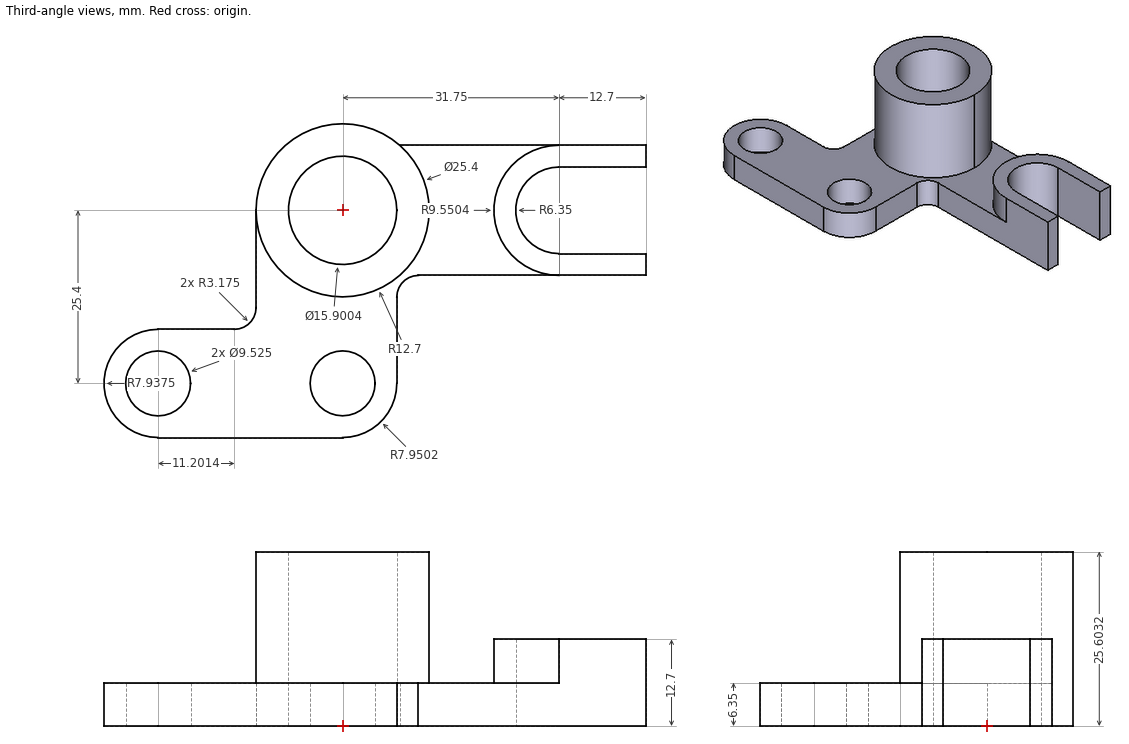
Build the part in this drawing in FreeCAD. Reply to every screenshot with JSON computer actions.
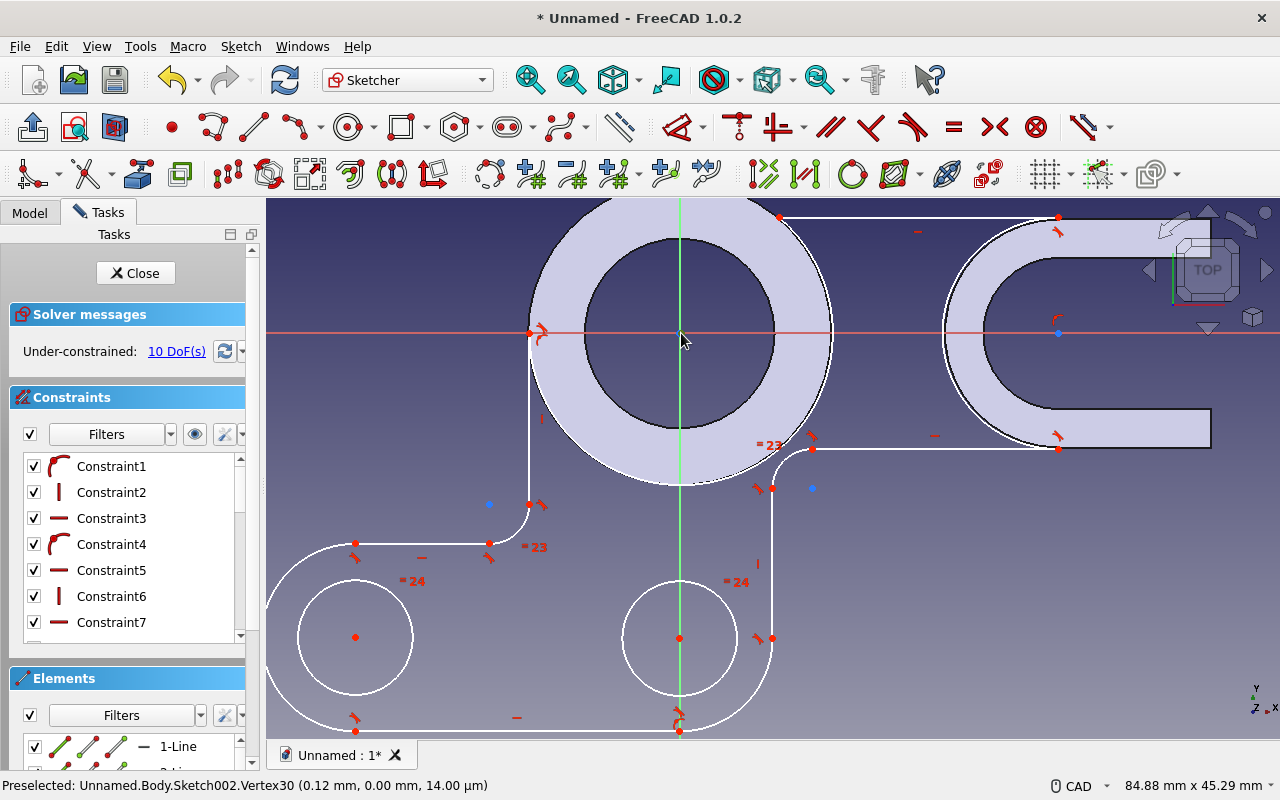
{"action": "left_click", "coordinate": [680, 538]}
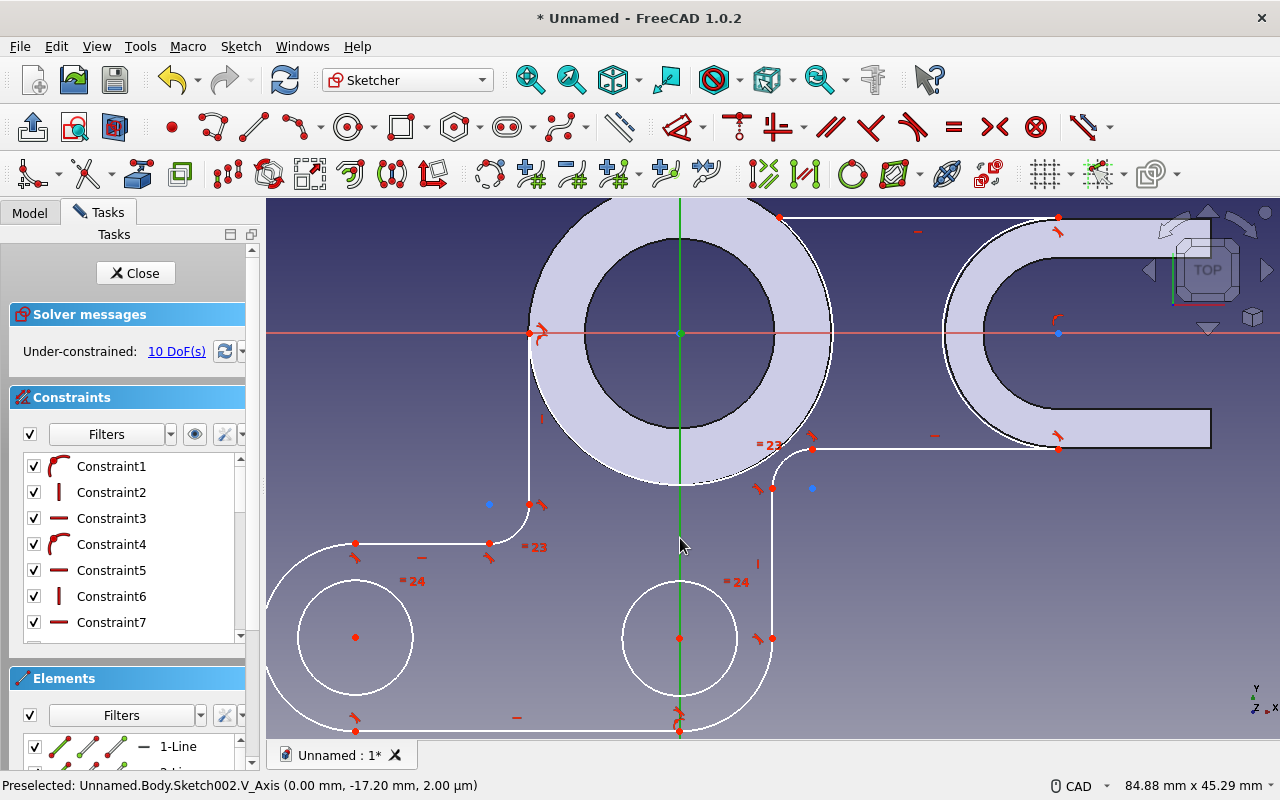
{"action": "left_click", "coordinate": [737, 128]}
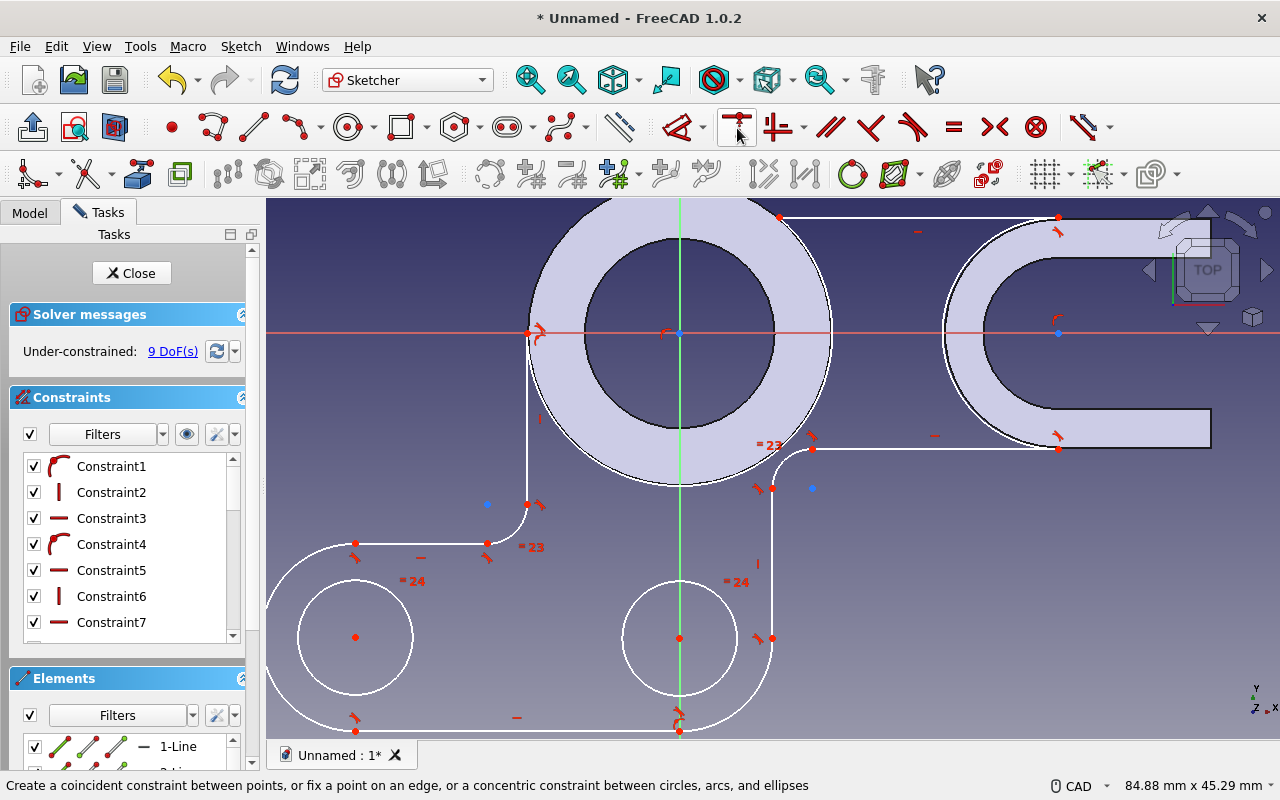
{"action": "left_click", "coordinate": [676, 128]}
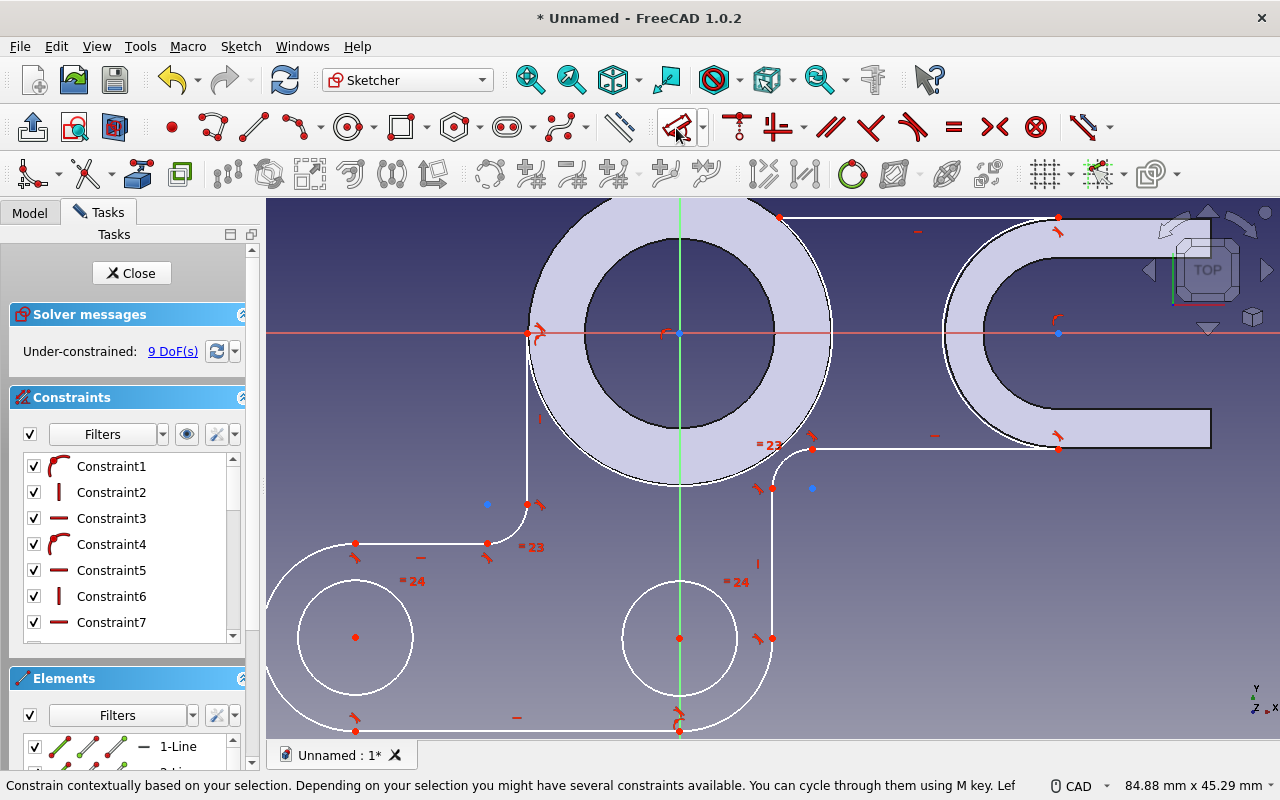
{"action": "left_click", "coordinate": [505, 540]}
{"action": "left_click", "coordinate": [519, 569]}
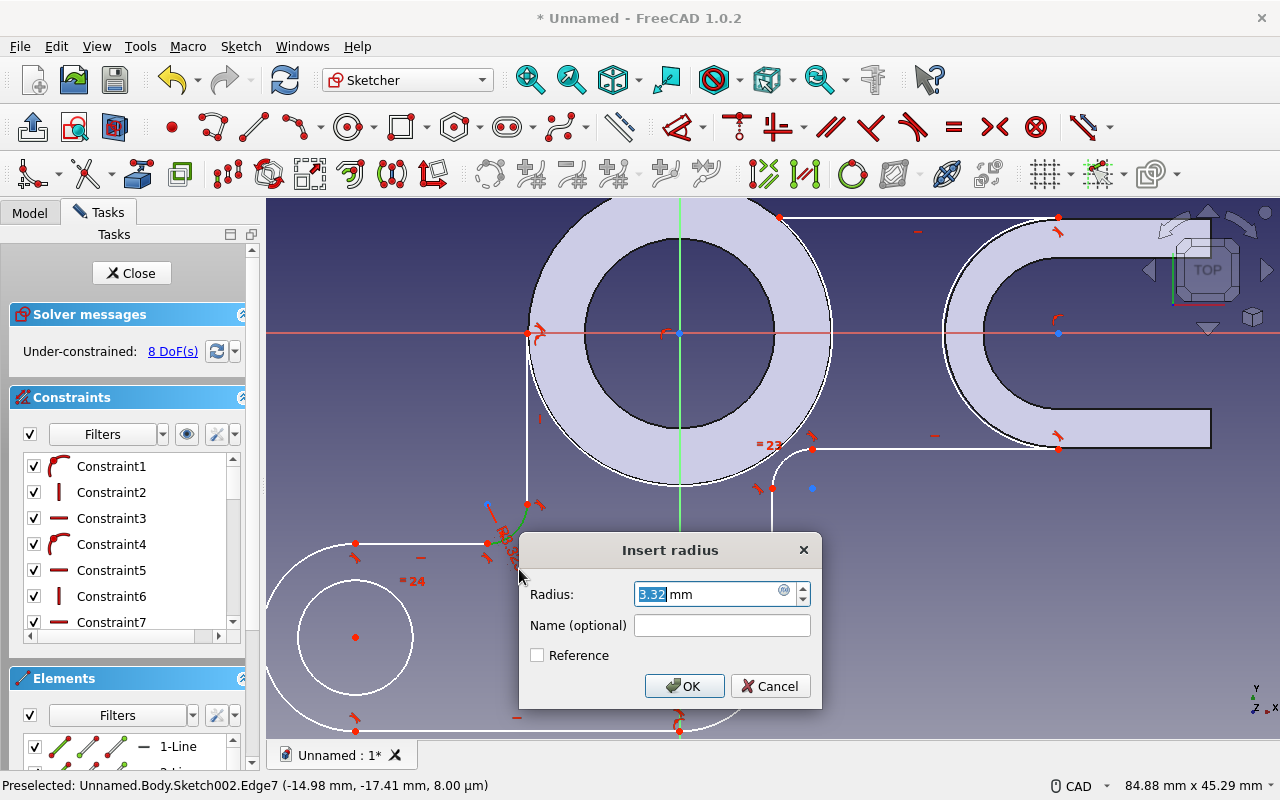
{"action": "type", "text": "3.175"}
{"action": "key", "text": "Return"}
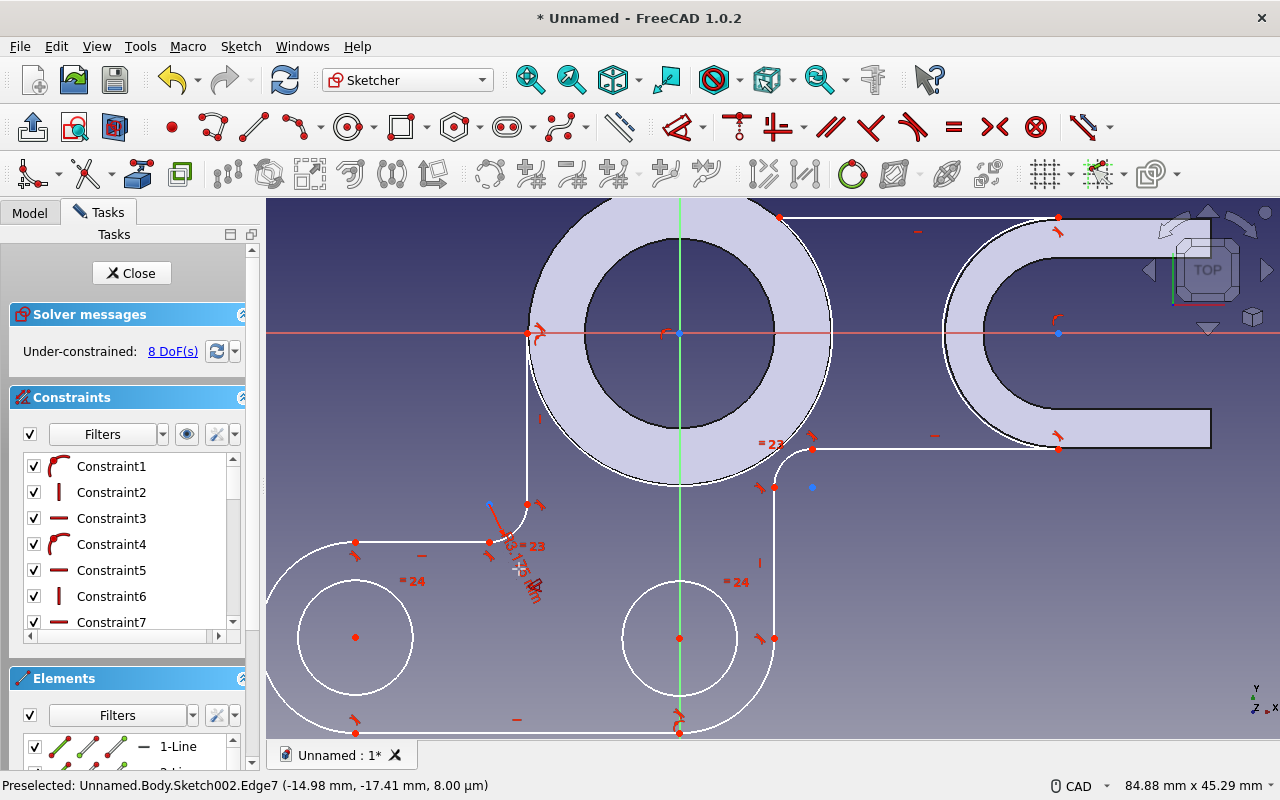
{"action": "left_click", "coordinate": [299, 560]}
{"action": "left_click", "coordinate": [339, 511]}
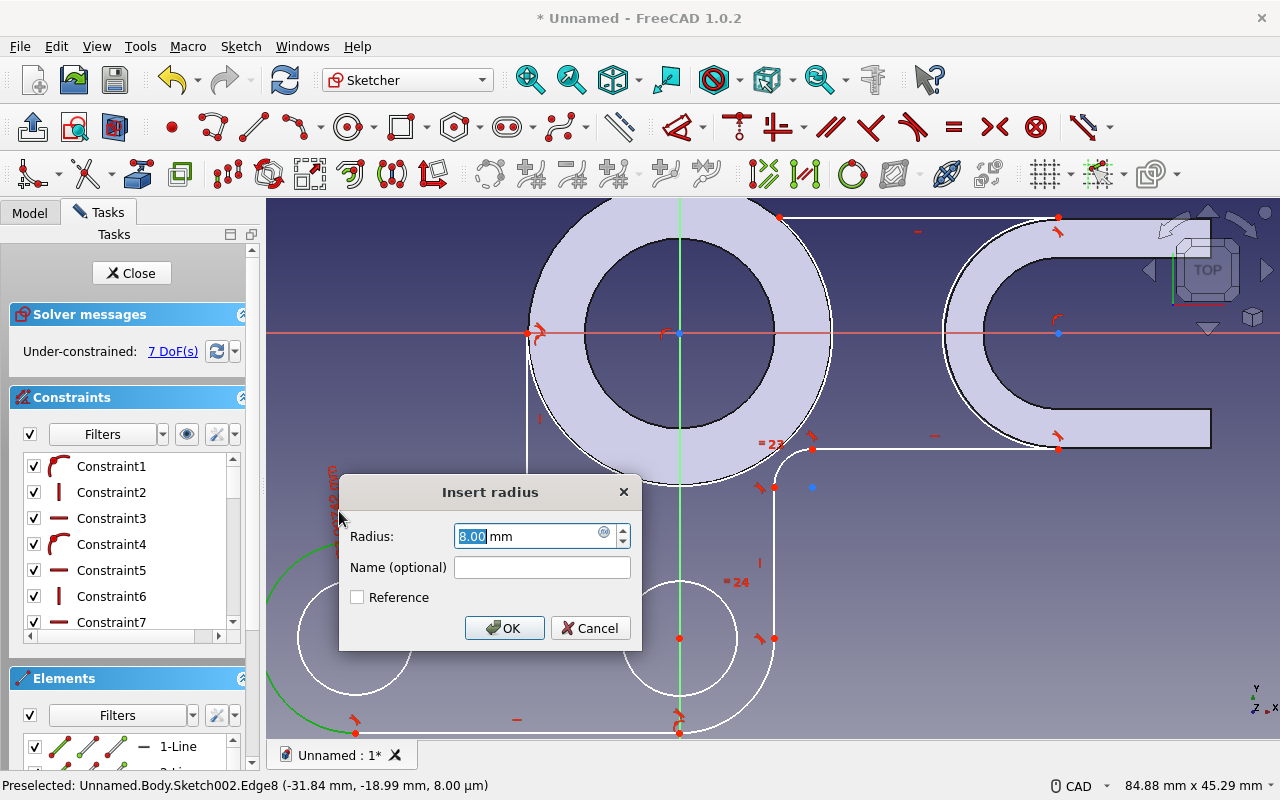
{"action": "type", "text": "7.9375"}
{"action": "key", "text": "Return"}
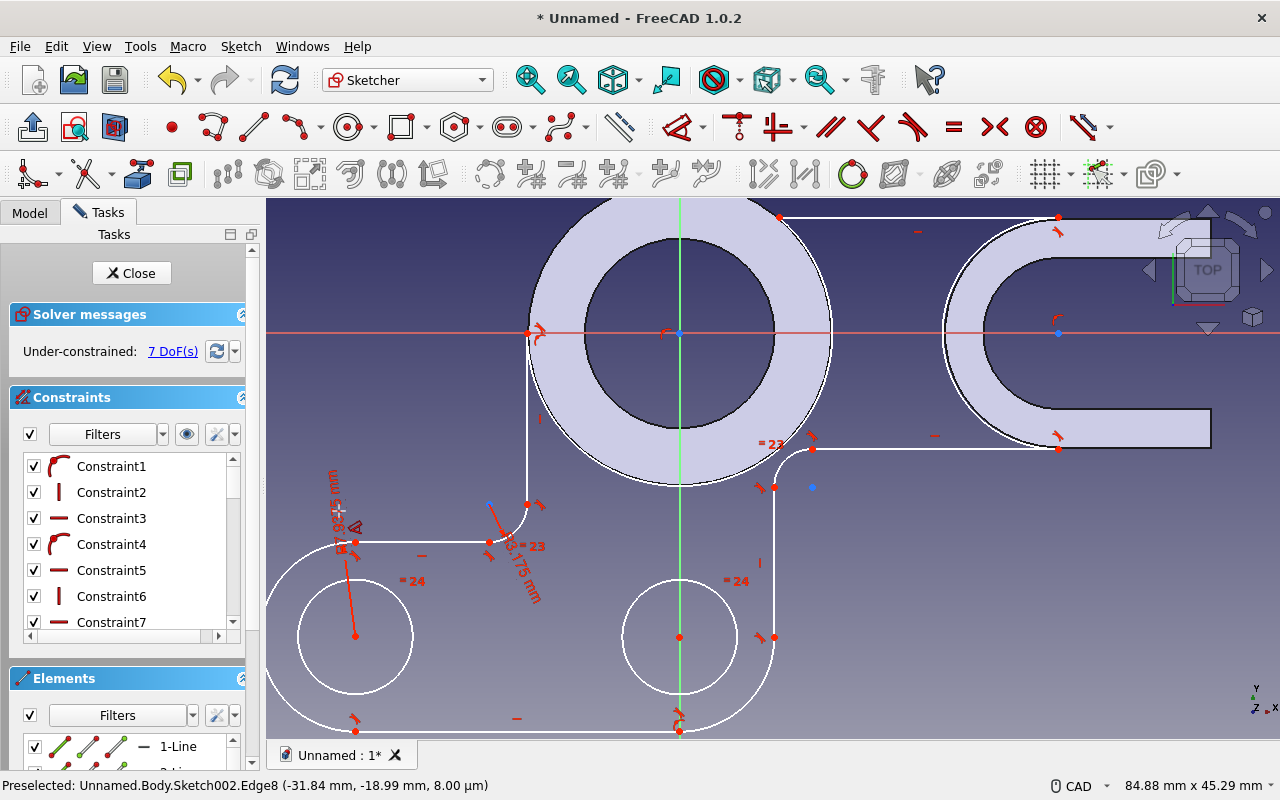
{"action": "left_click", "coordinate": [764, 680]}
{"action": "left_click", "coordinate": [793, 694]}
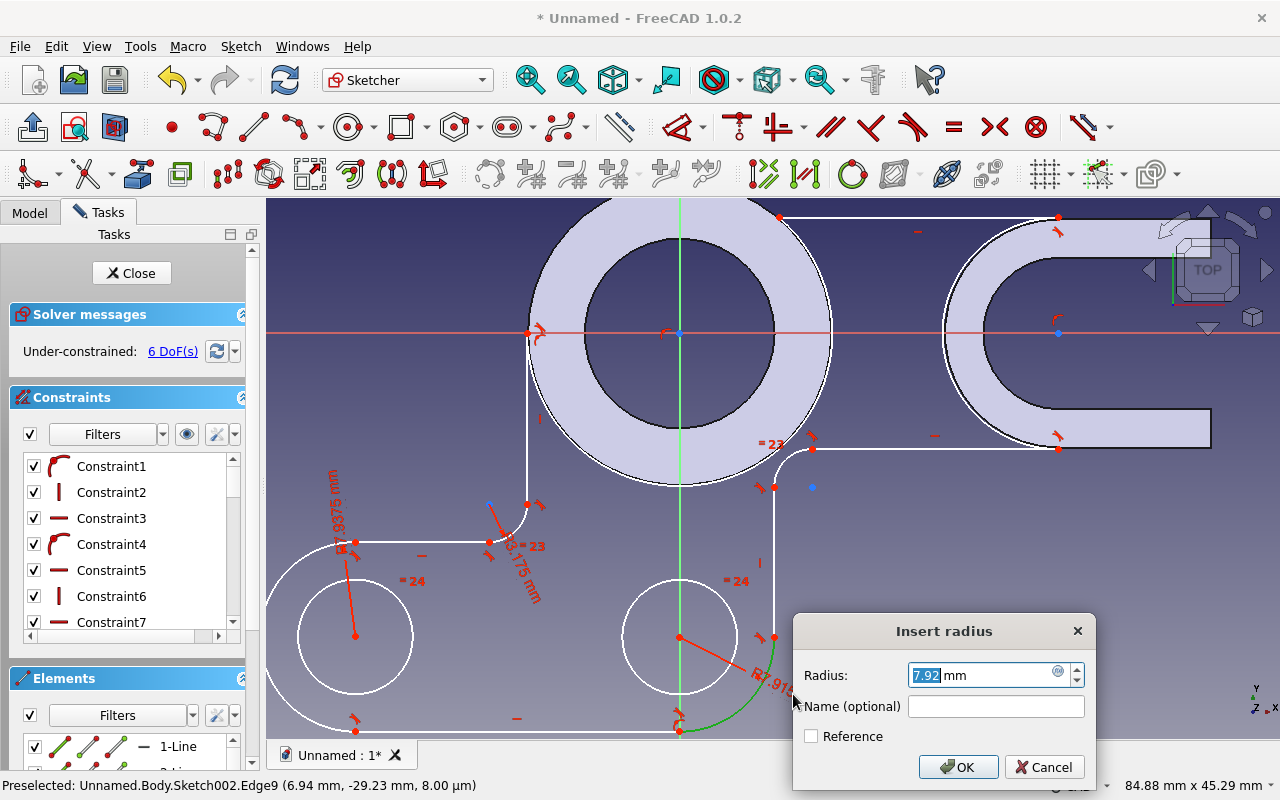
{"action": "type", "text": "7.9502"}
{"action": "key", "text": "Return"}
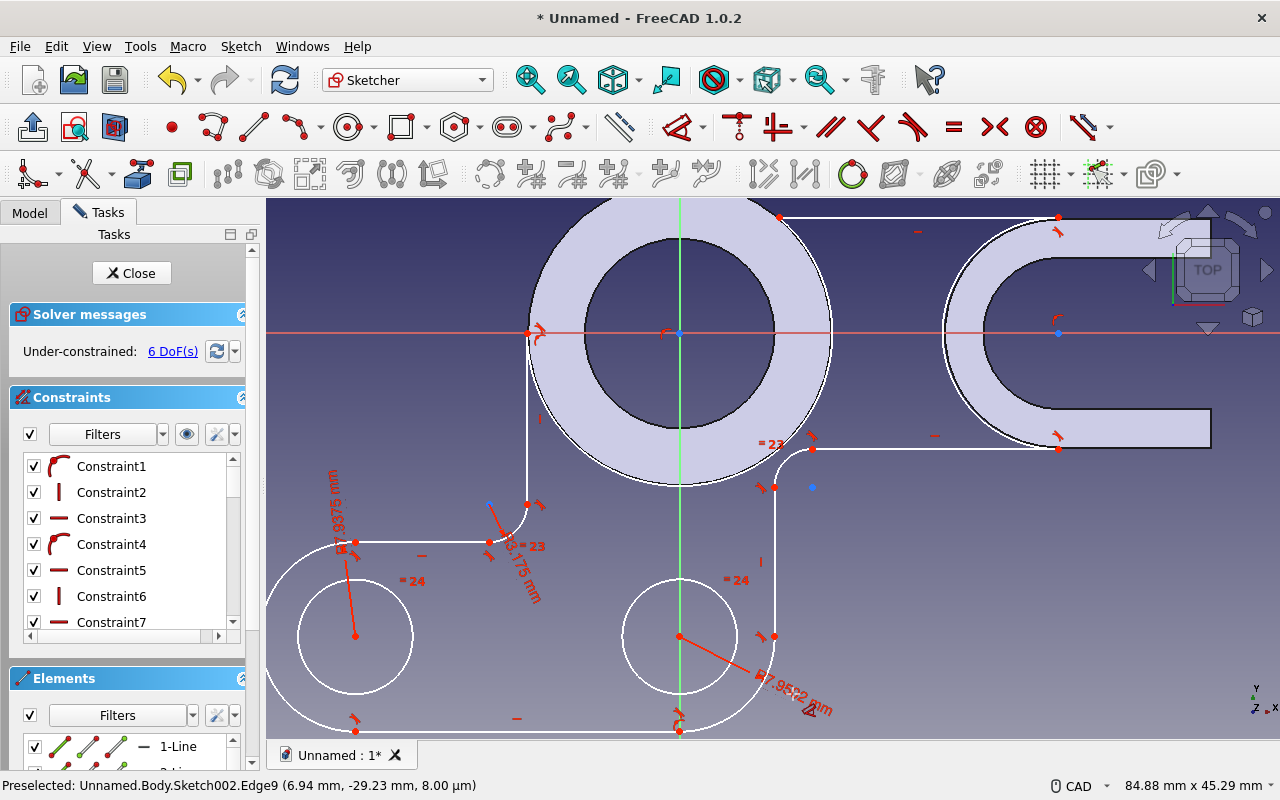
{"action": "left_click", "coordinate": [965, 266]}
{"action": "left_click", "coordinate": [939, 247]}